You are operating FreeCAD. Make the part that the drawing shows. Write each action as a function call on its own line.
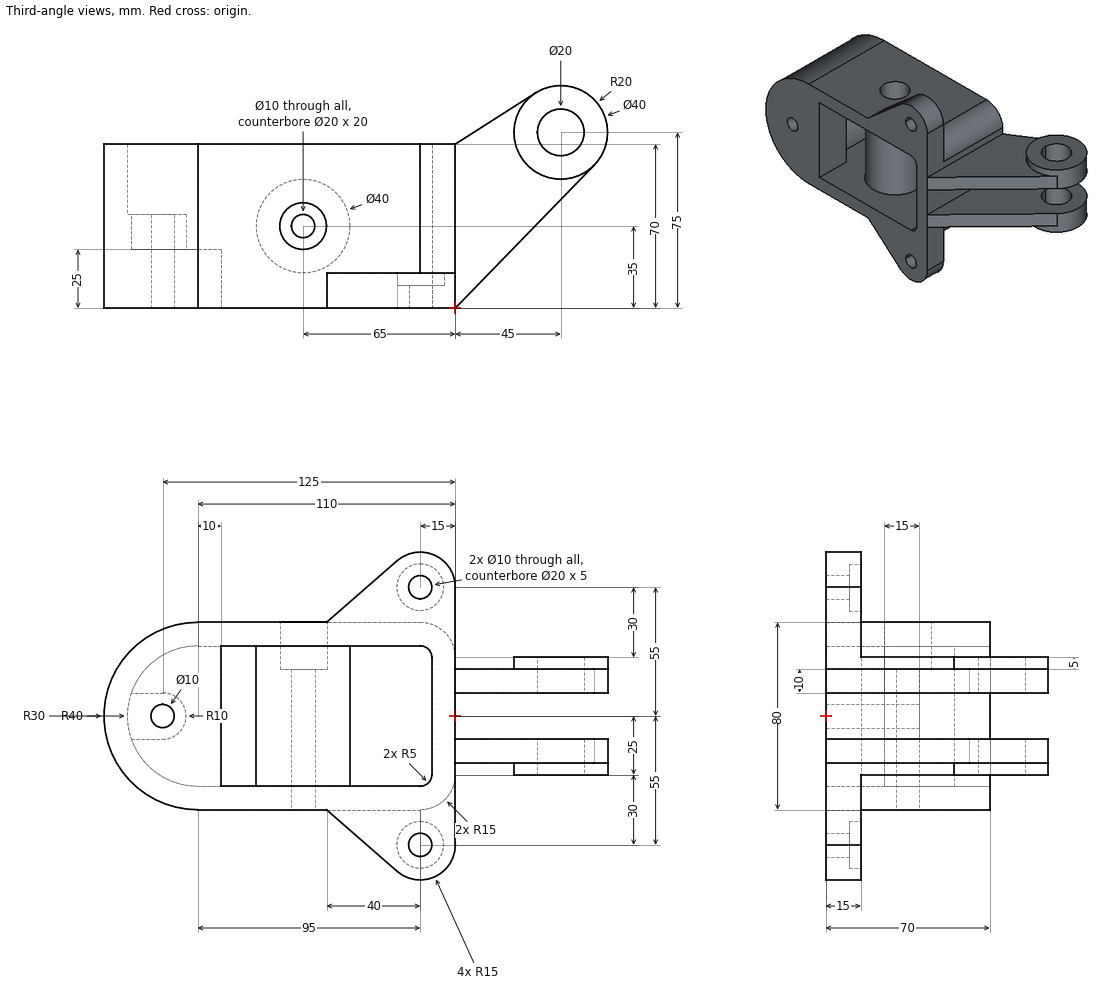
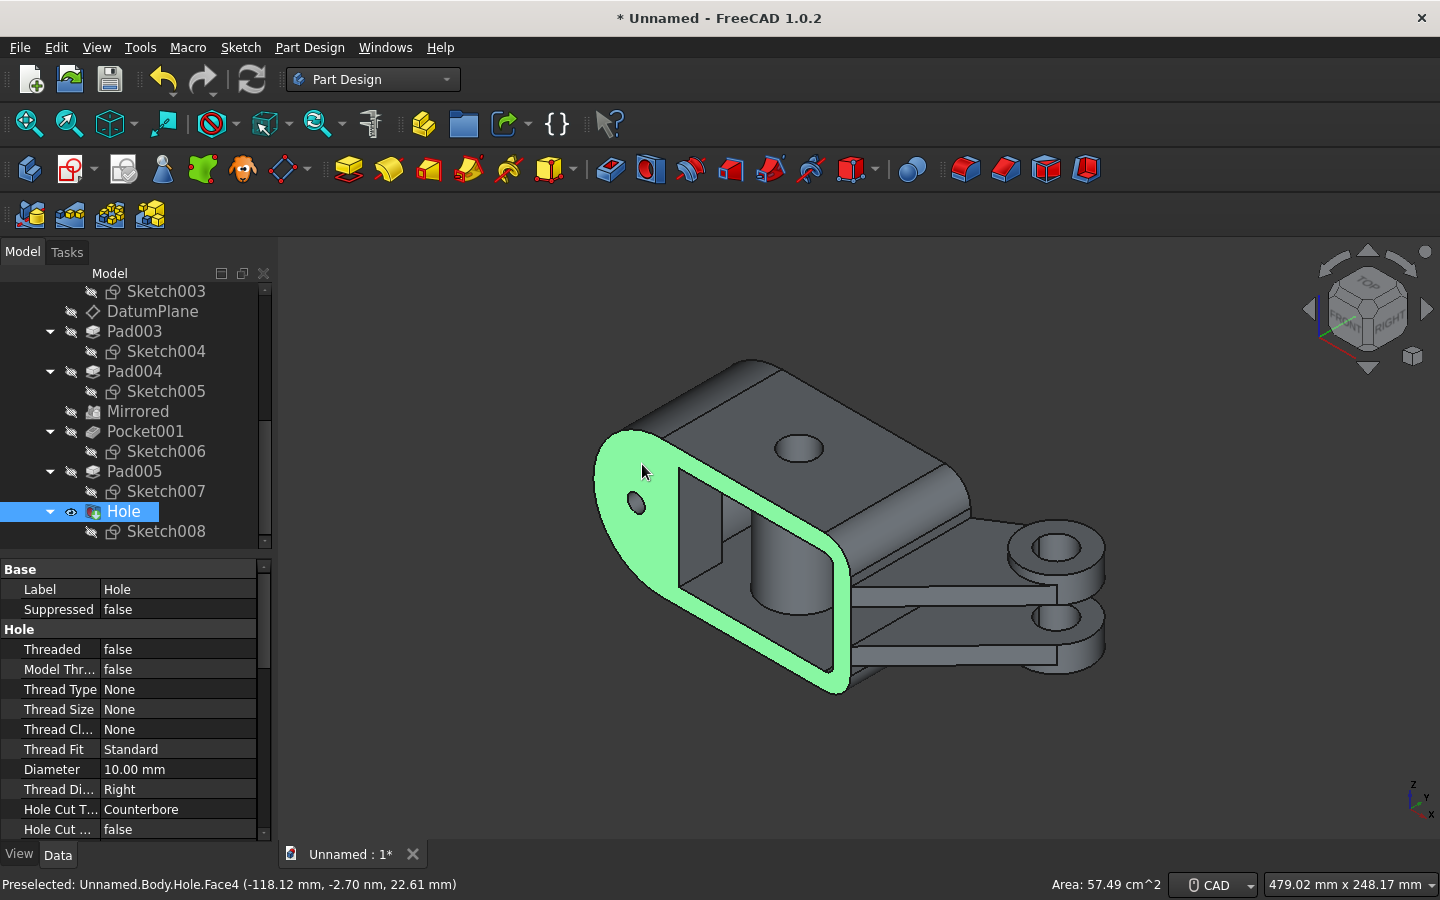
click(70, 170)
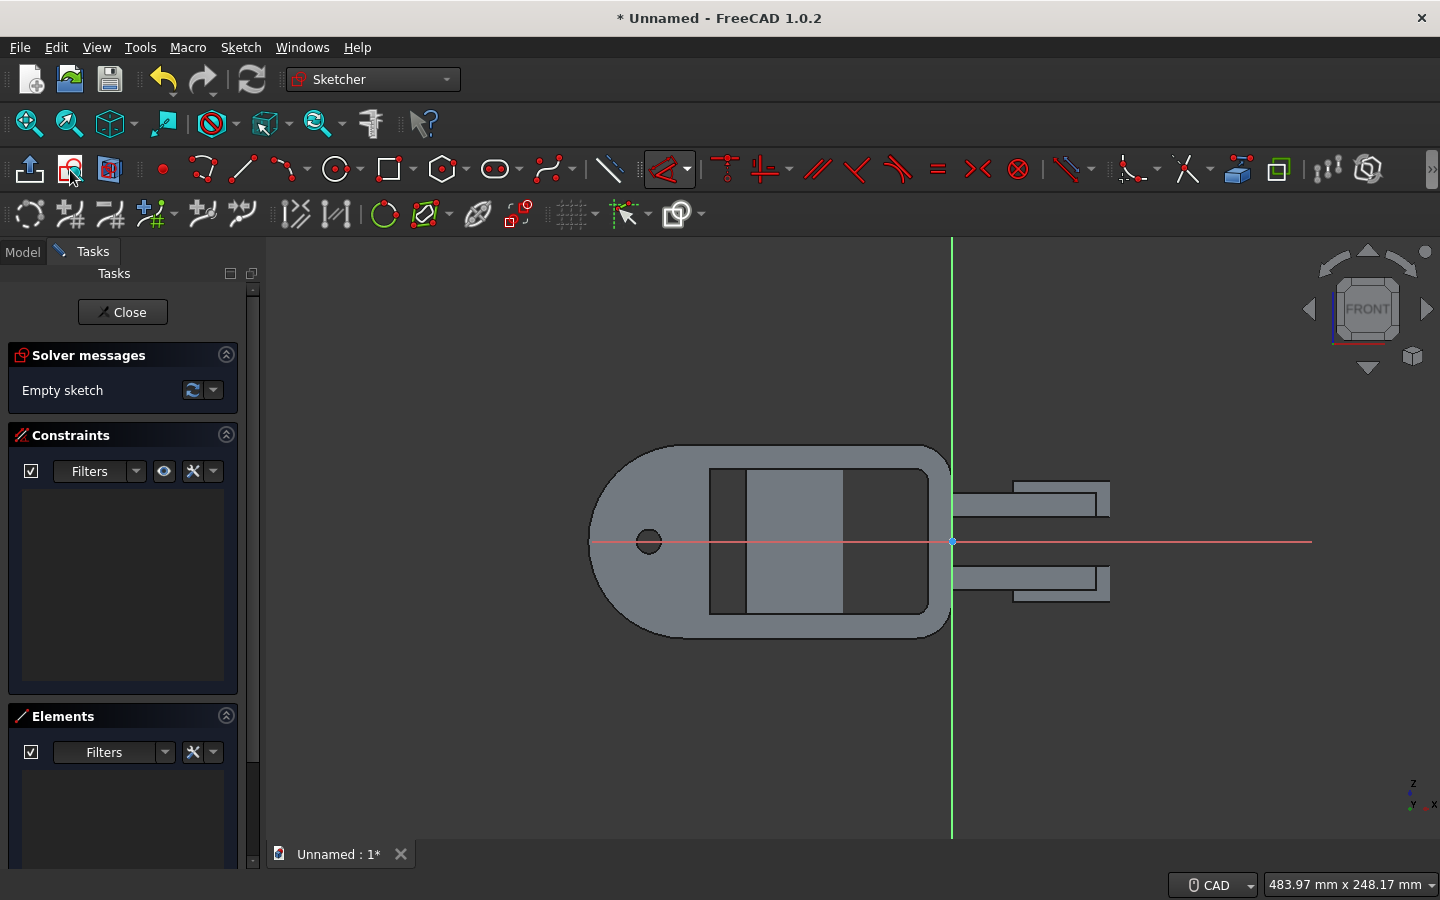
key(g)
key(l)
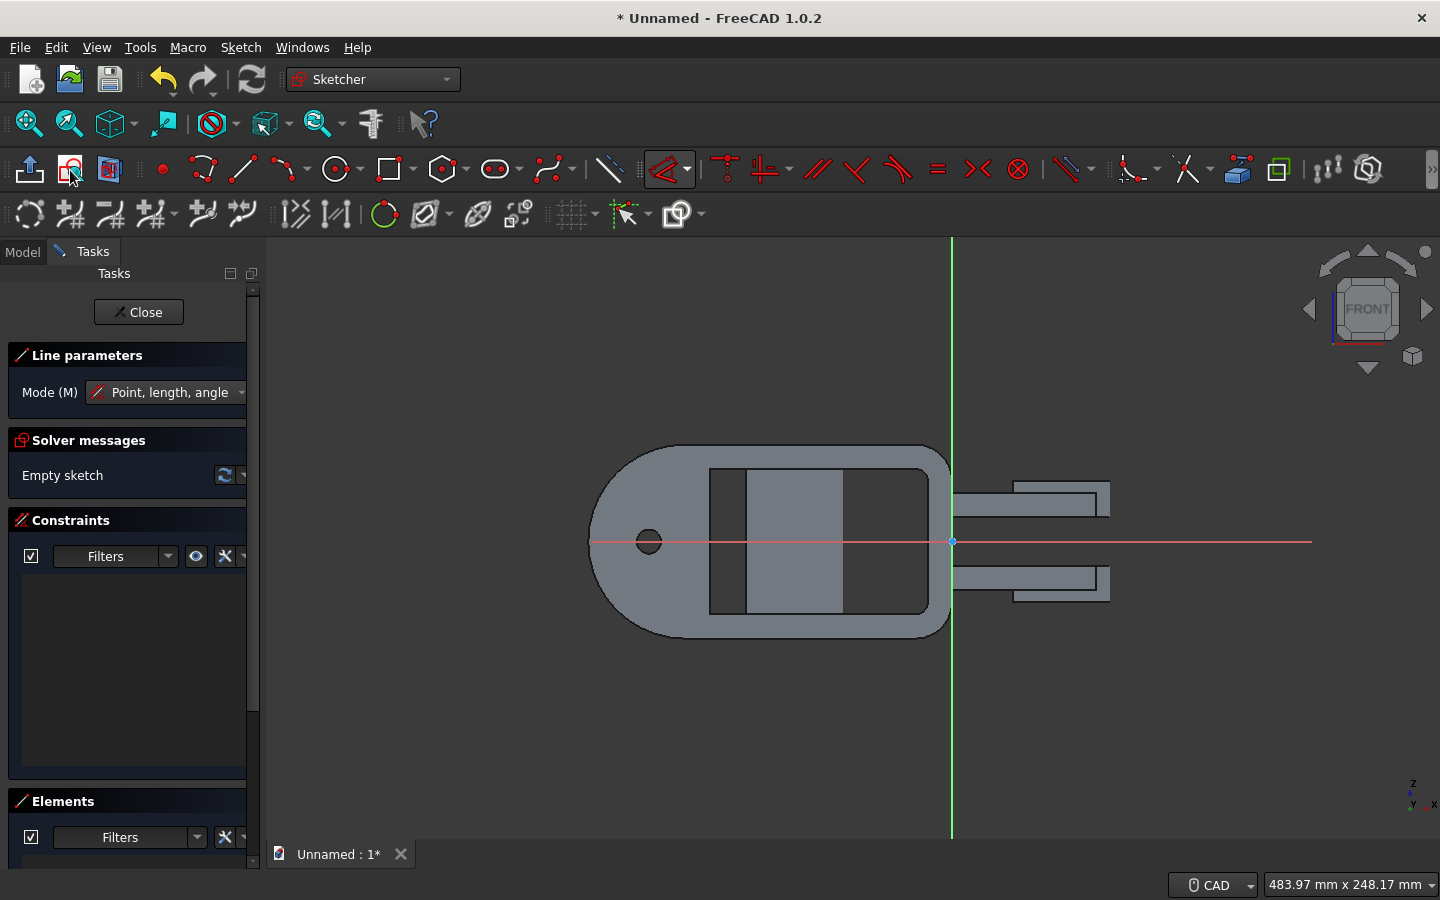
click(952, 602)
click(943, 675)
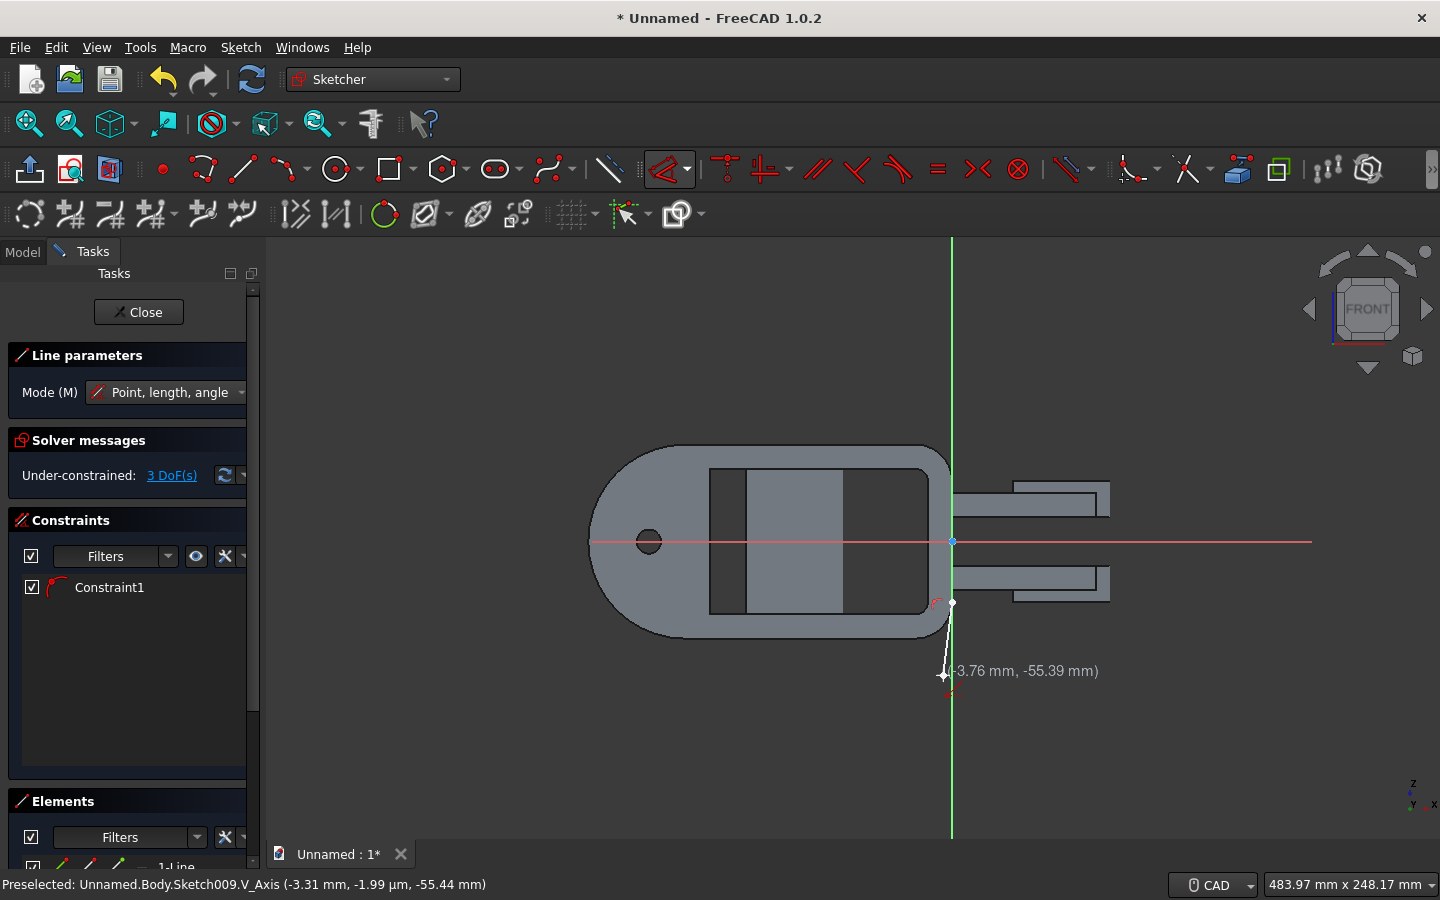
key(g)
key(m)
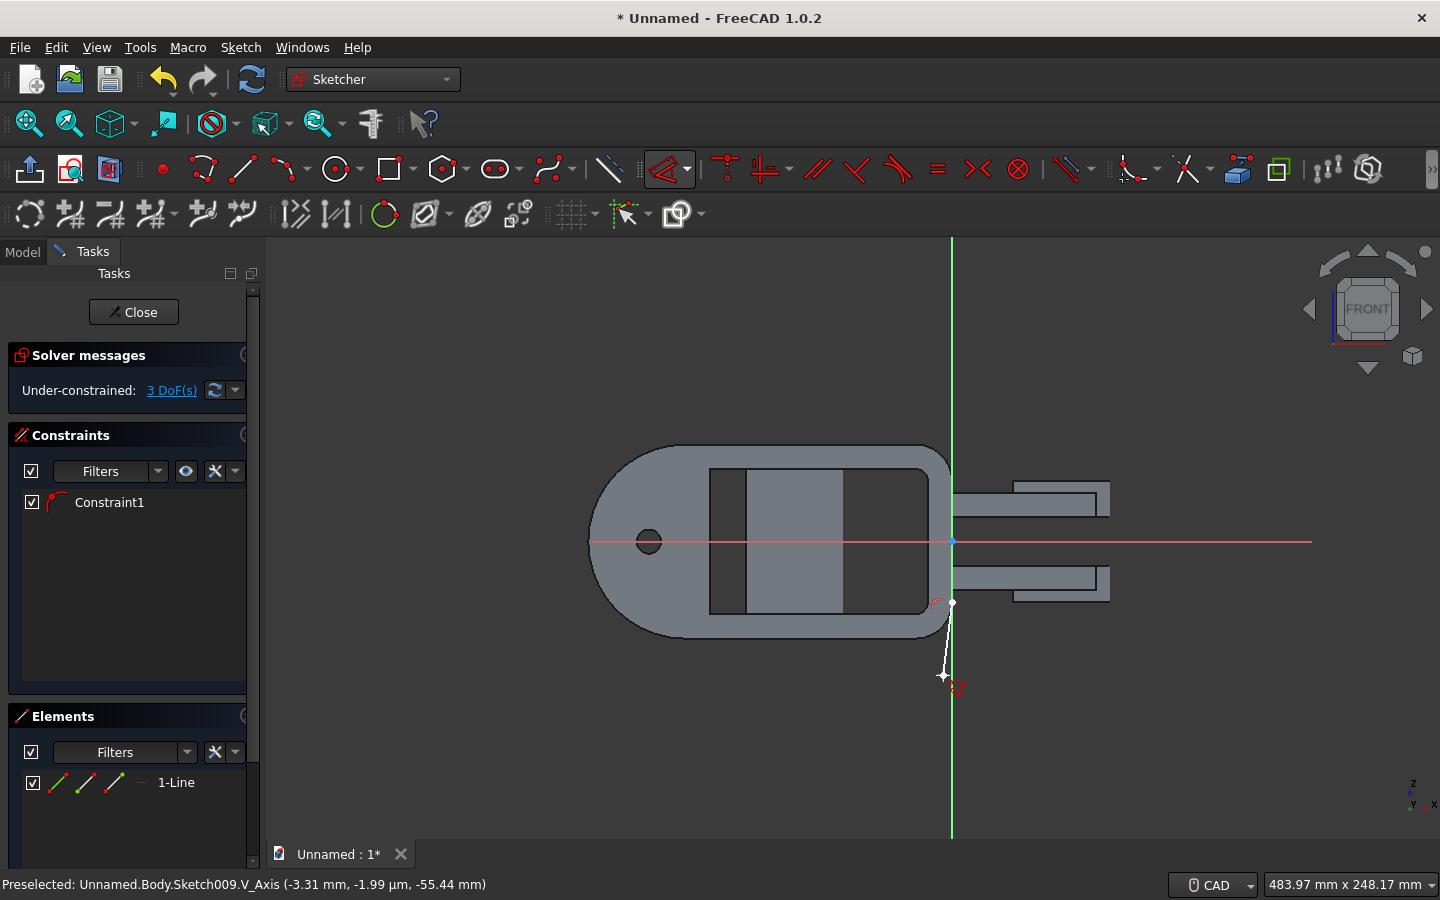
click(892, 702)
click(819, 639)
click(916, 639)
right_click(916, 639)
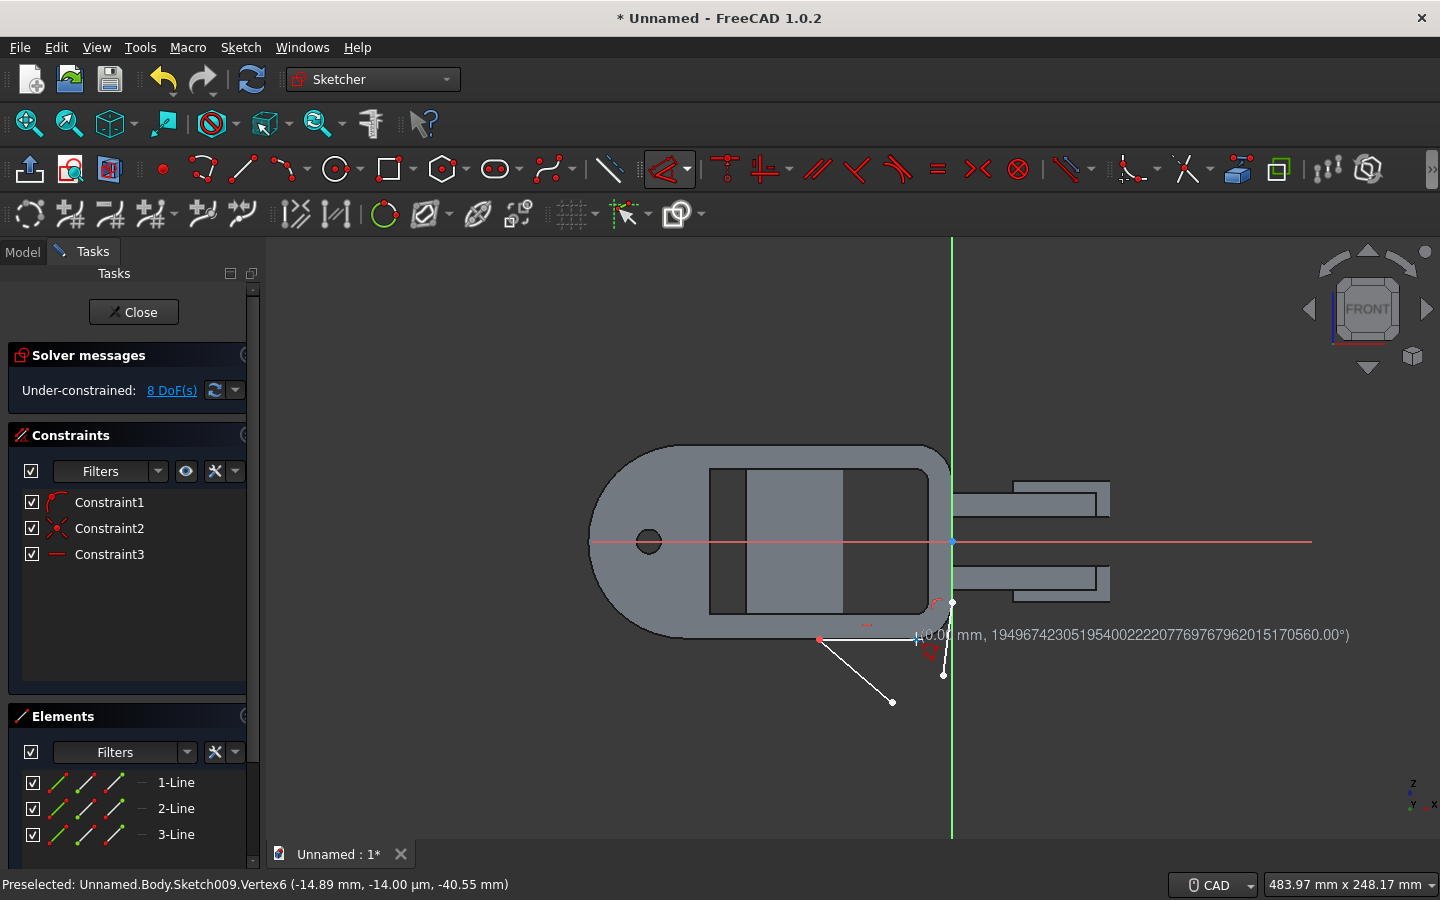
key(g)
key(3)
key(a)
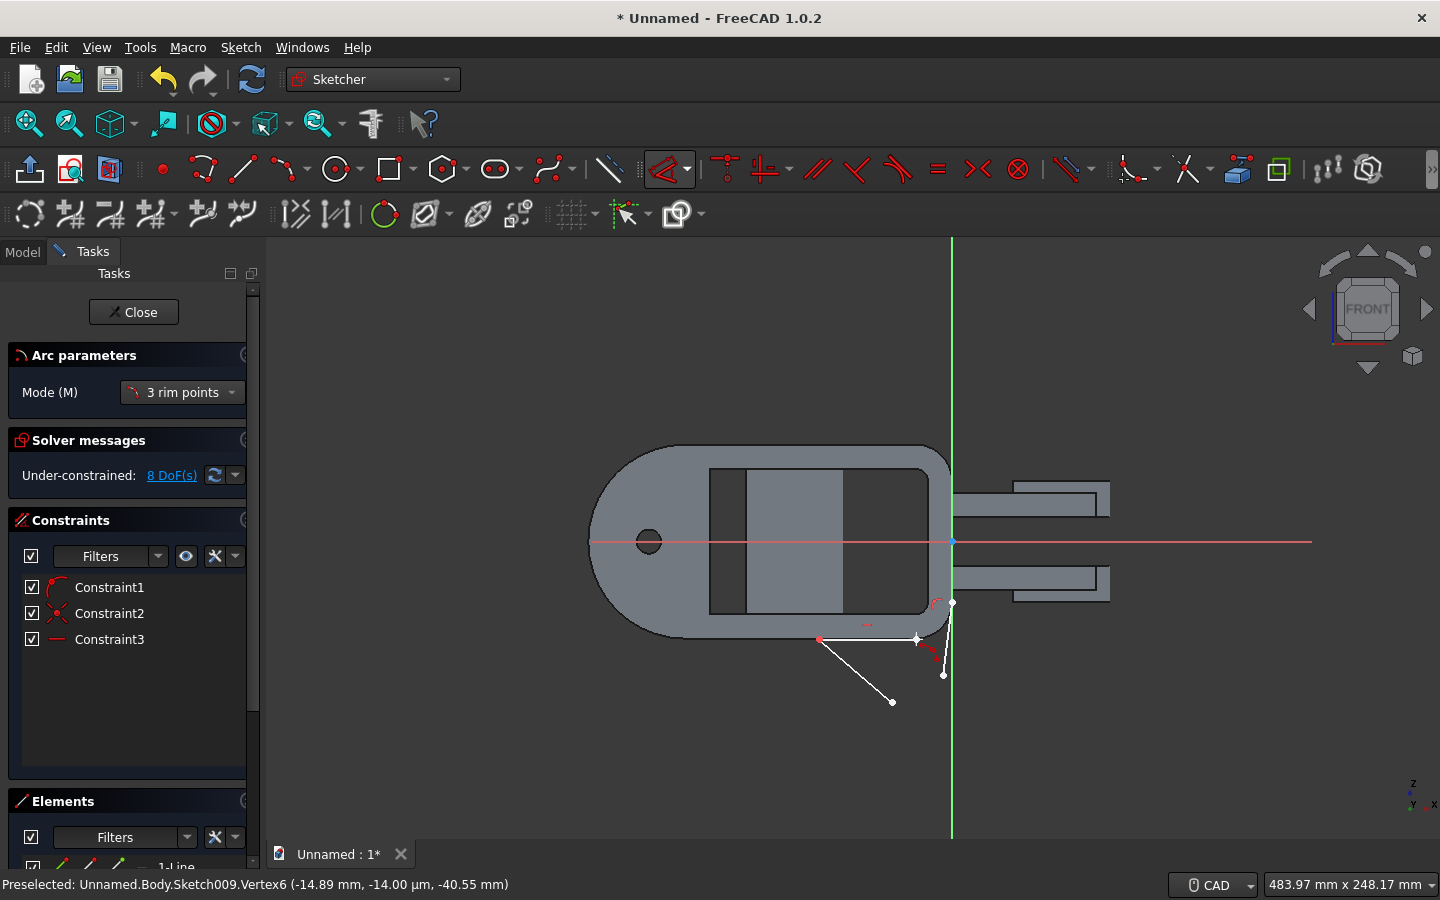
click(943, 676)
click(892, 703)
click(931, 708)